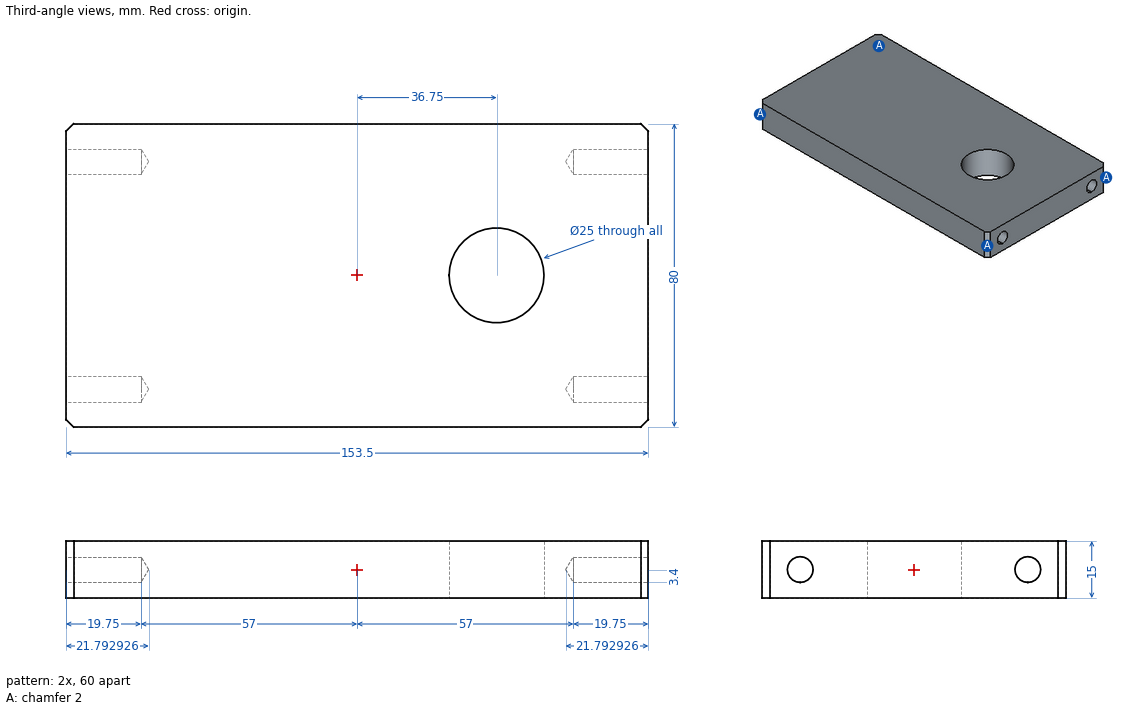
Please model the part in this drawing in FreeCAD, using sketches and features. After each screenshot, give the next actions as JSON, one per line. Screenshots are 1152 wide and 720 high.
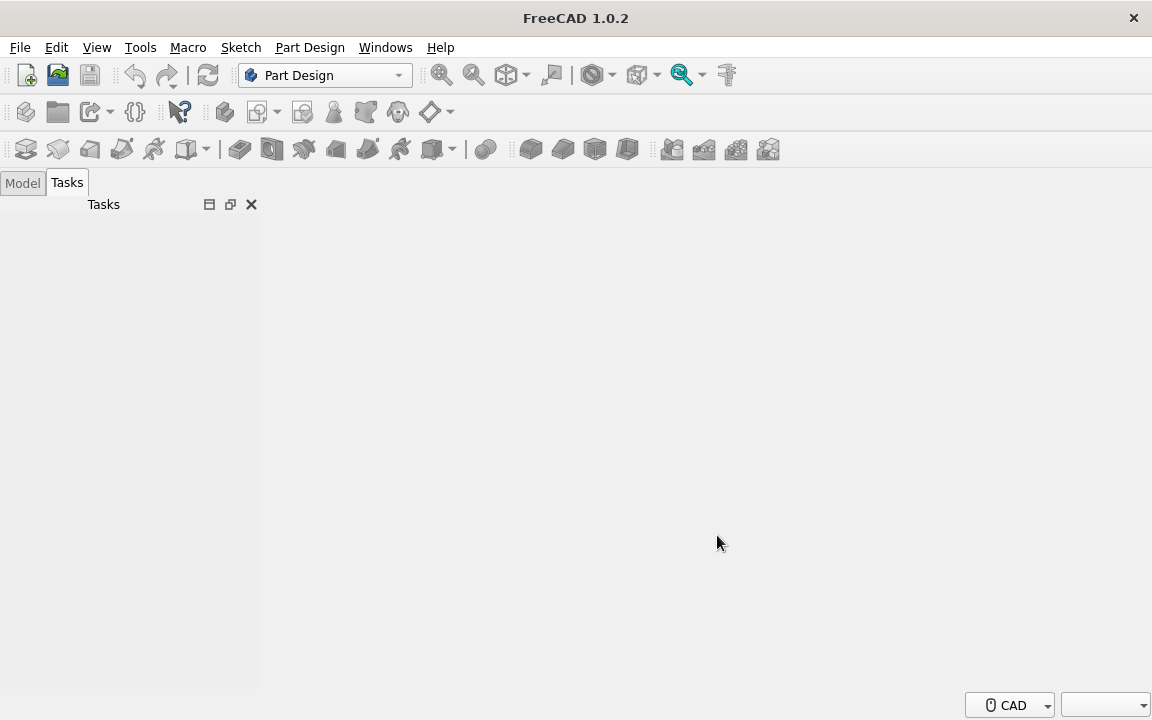
{"action": "key", "text": "ctrl+n"}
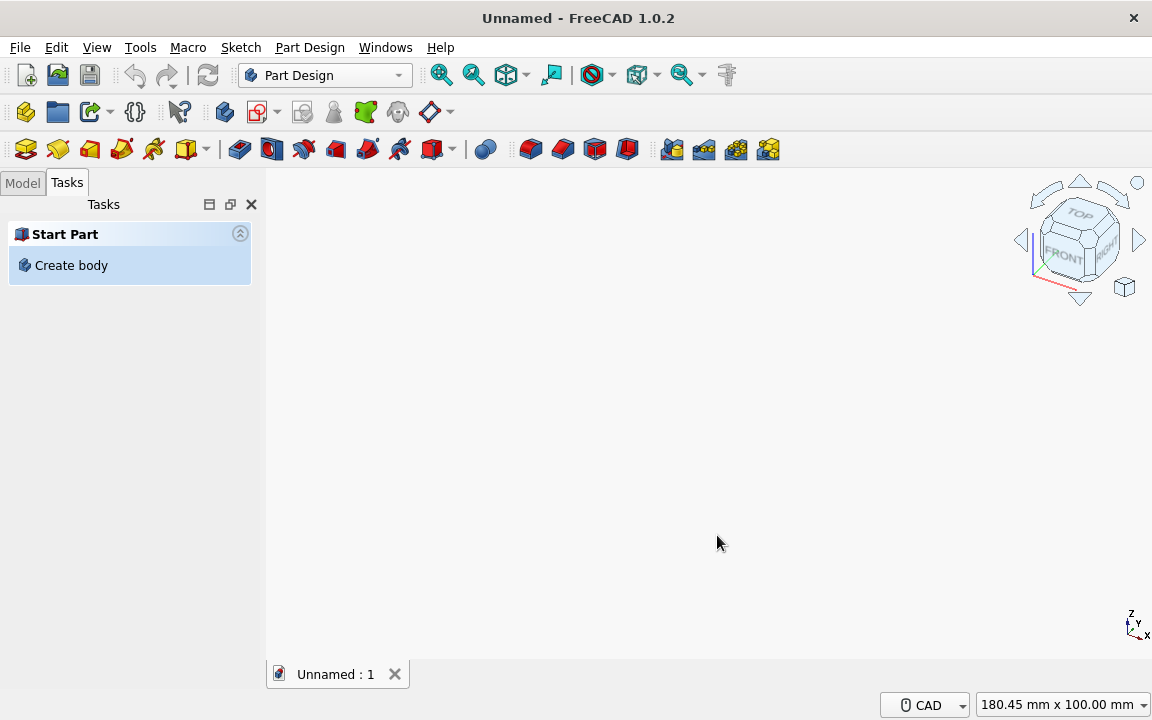
{"action": "left_click", "coordinate": [258, 112]}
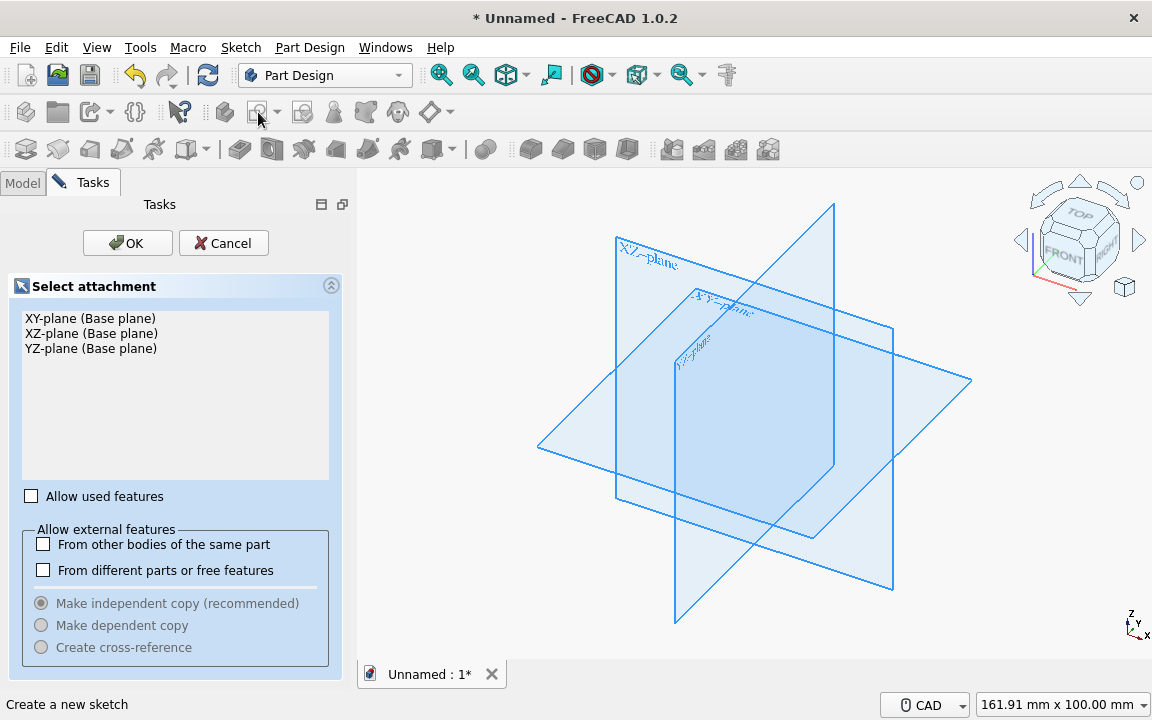
{"action": "left_click", "coordinate": [82, 318]}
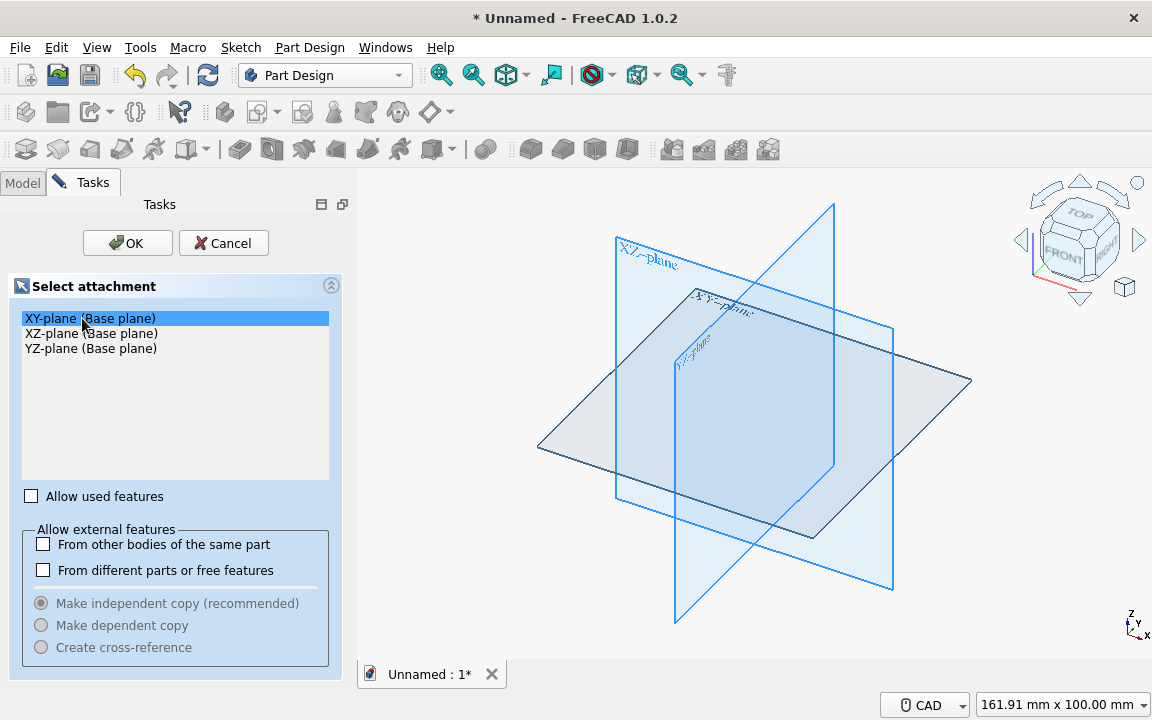
{"action": "left_click", "coordinate": [128, 243]}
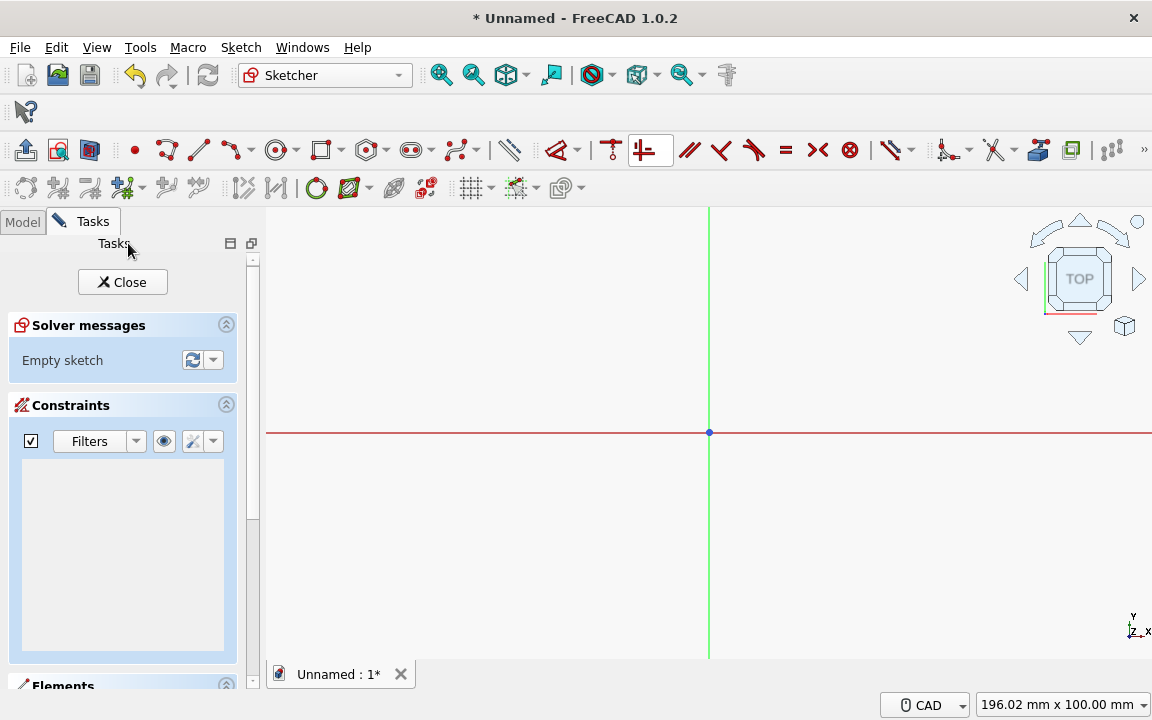
{"action": "scroll", "coordinate": [501, 433], "scroll_direction": "down", "scroll_amount": 2}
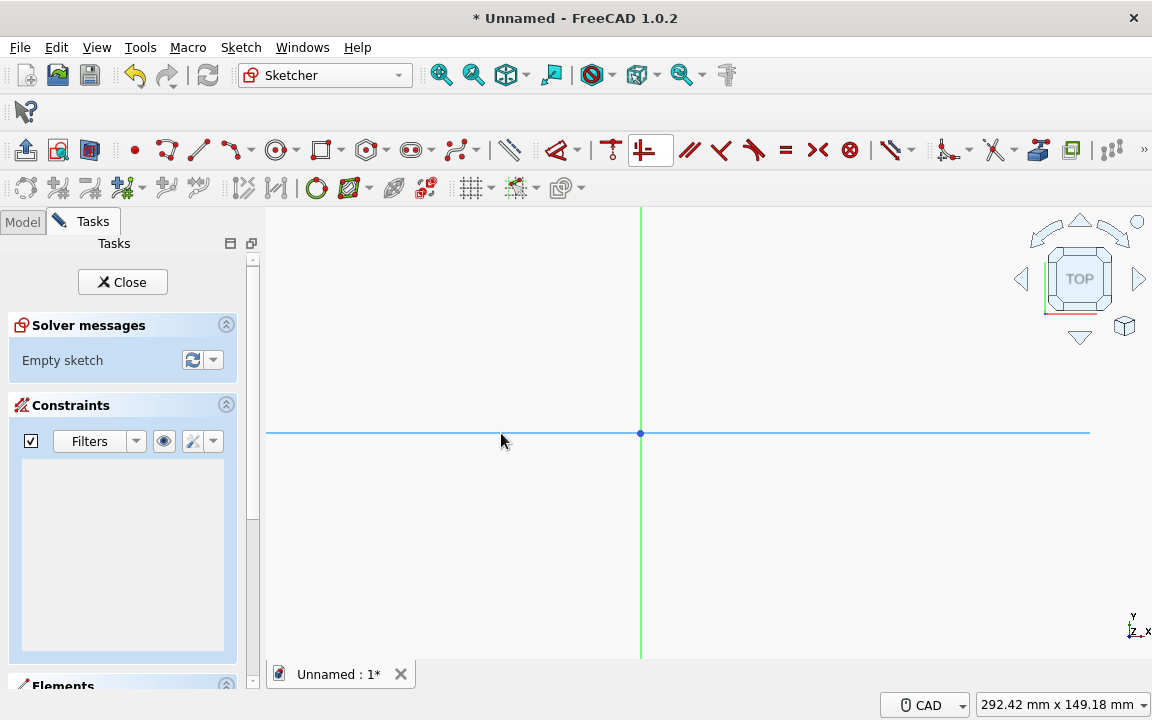
{"action": "key", "text": "g v"}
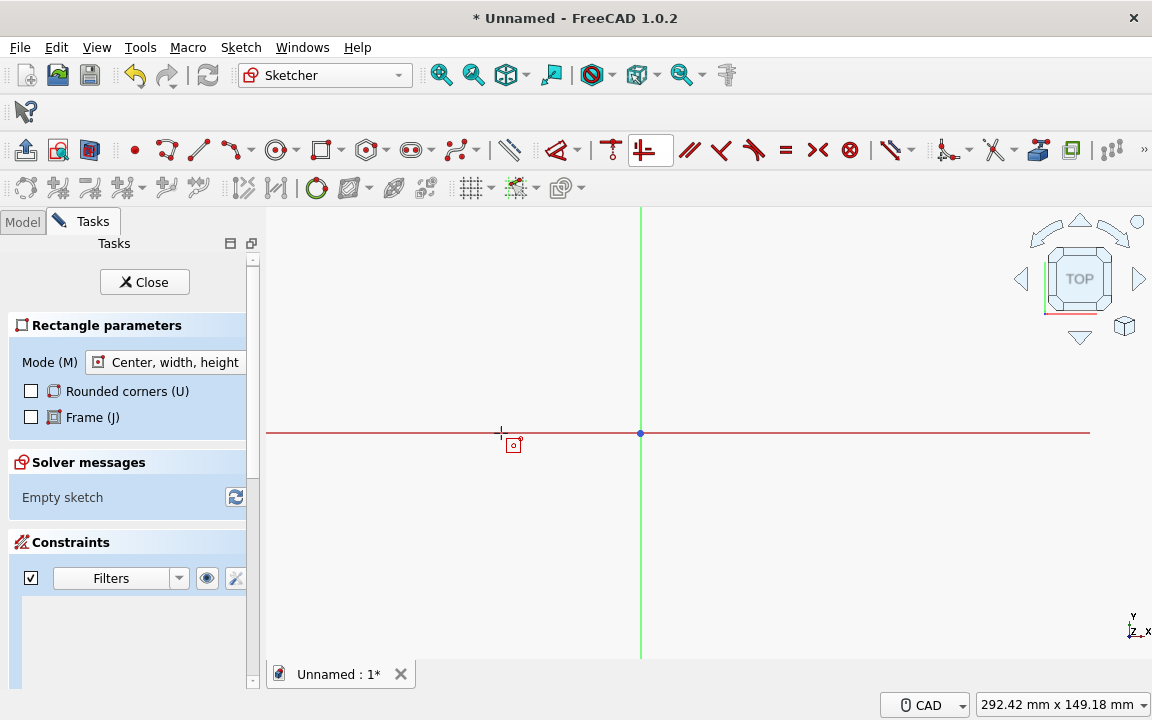
{"action": "left_click", "coordinate": [641, 433]}
{"action": "mouse_move", "coordinate": [873, 312]}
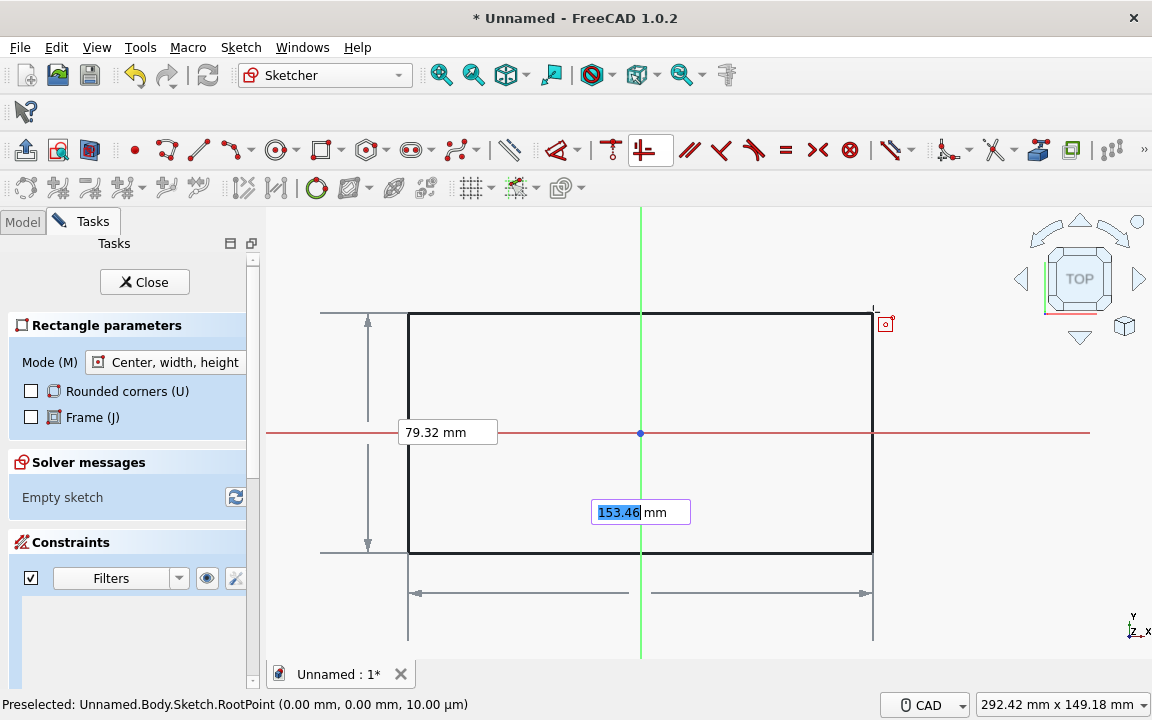
{"action": "type", "text": "153.5"}
{"action": "key", "text": "Tab"}
{"action": "type", "text": "80"}
{"action": "key", "text": "Return"}
{"action": "key", "text": "Escape"}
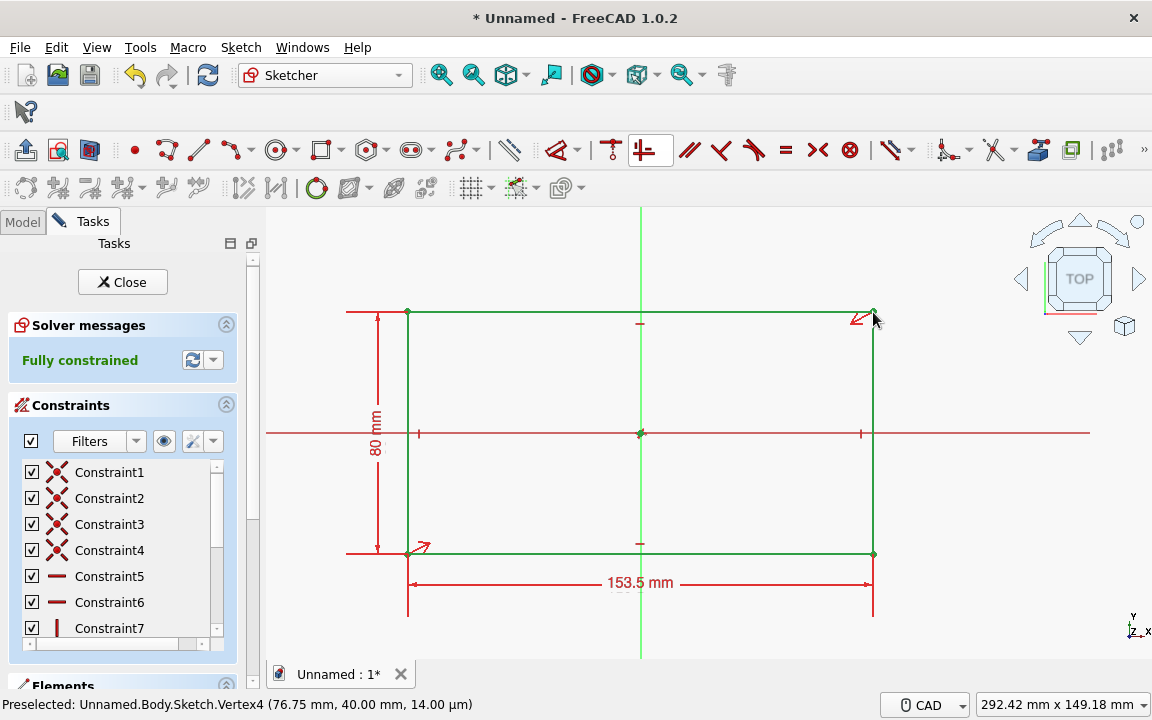
{"action": "left_click", "coordinate": [123, 282]}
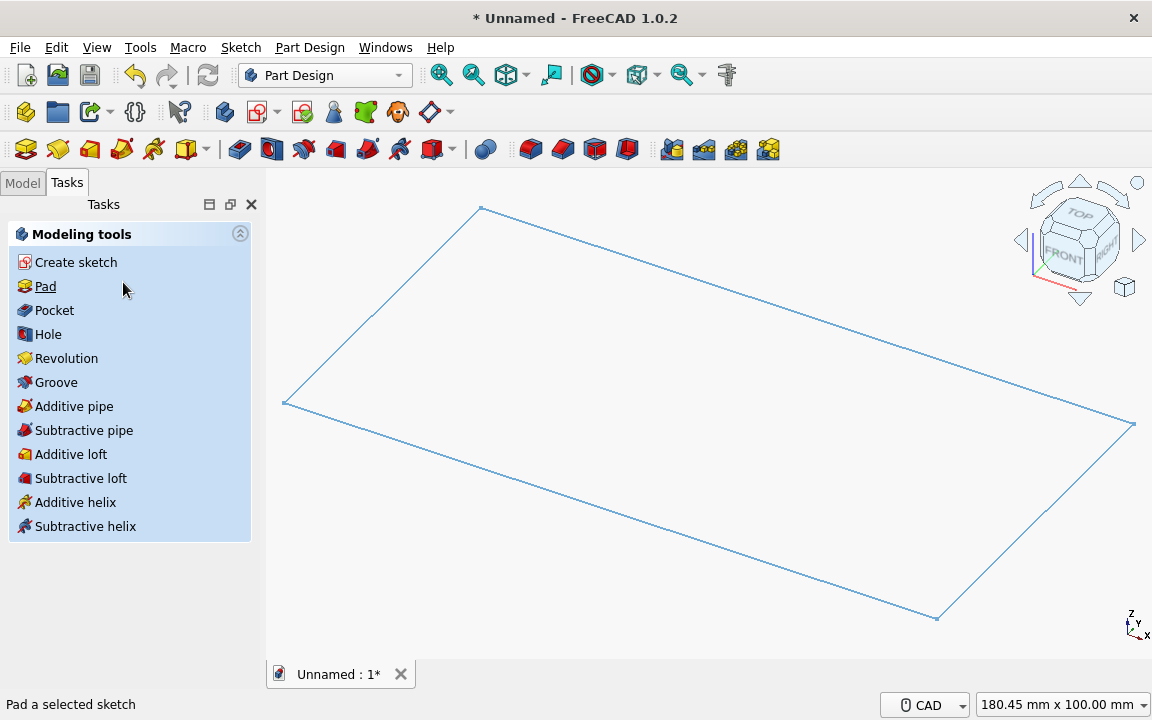
{"action": "left_click", "coordinate": [26, 150]}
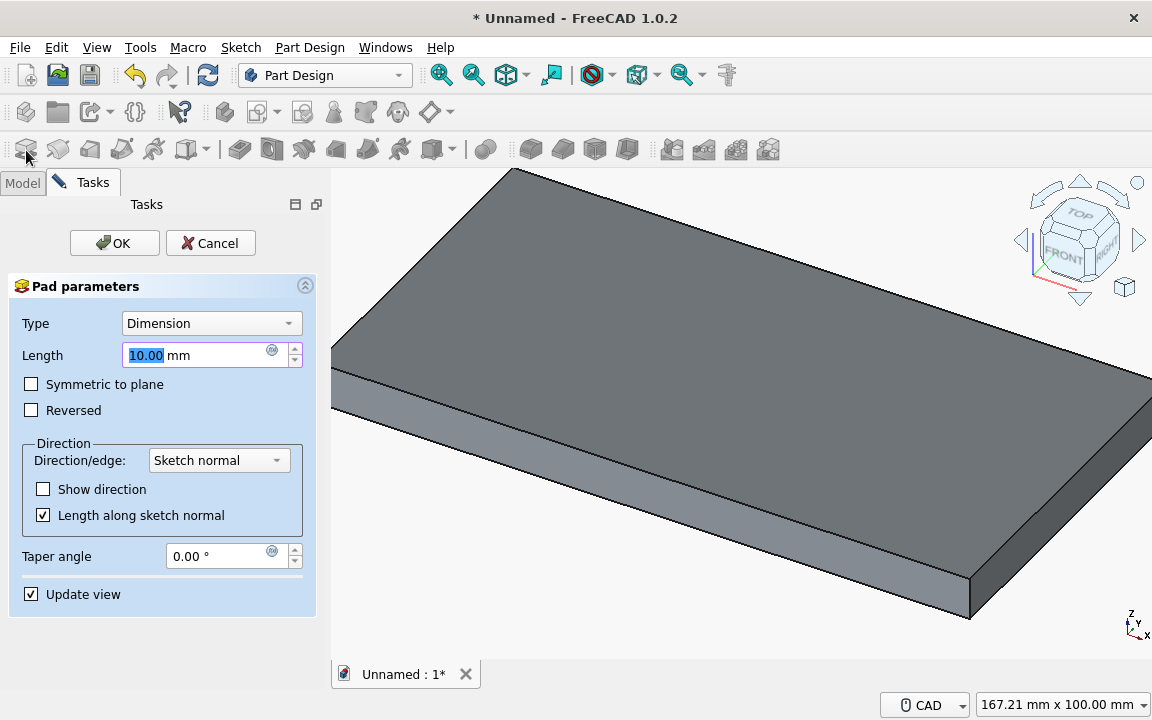
{"action": "type", "text": "15"}
{"action": "key", "text": "Tab"}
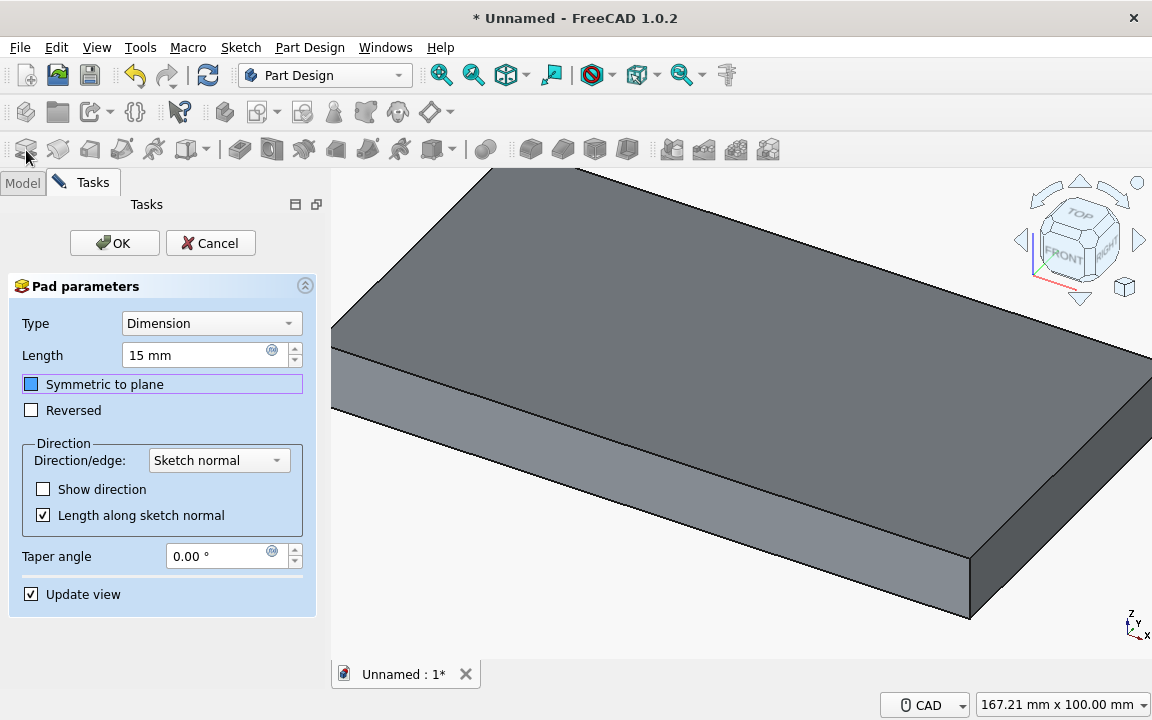
{"action": "left_click", "coordinate": [30, 384]}